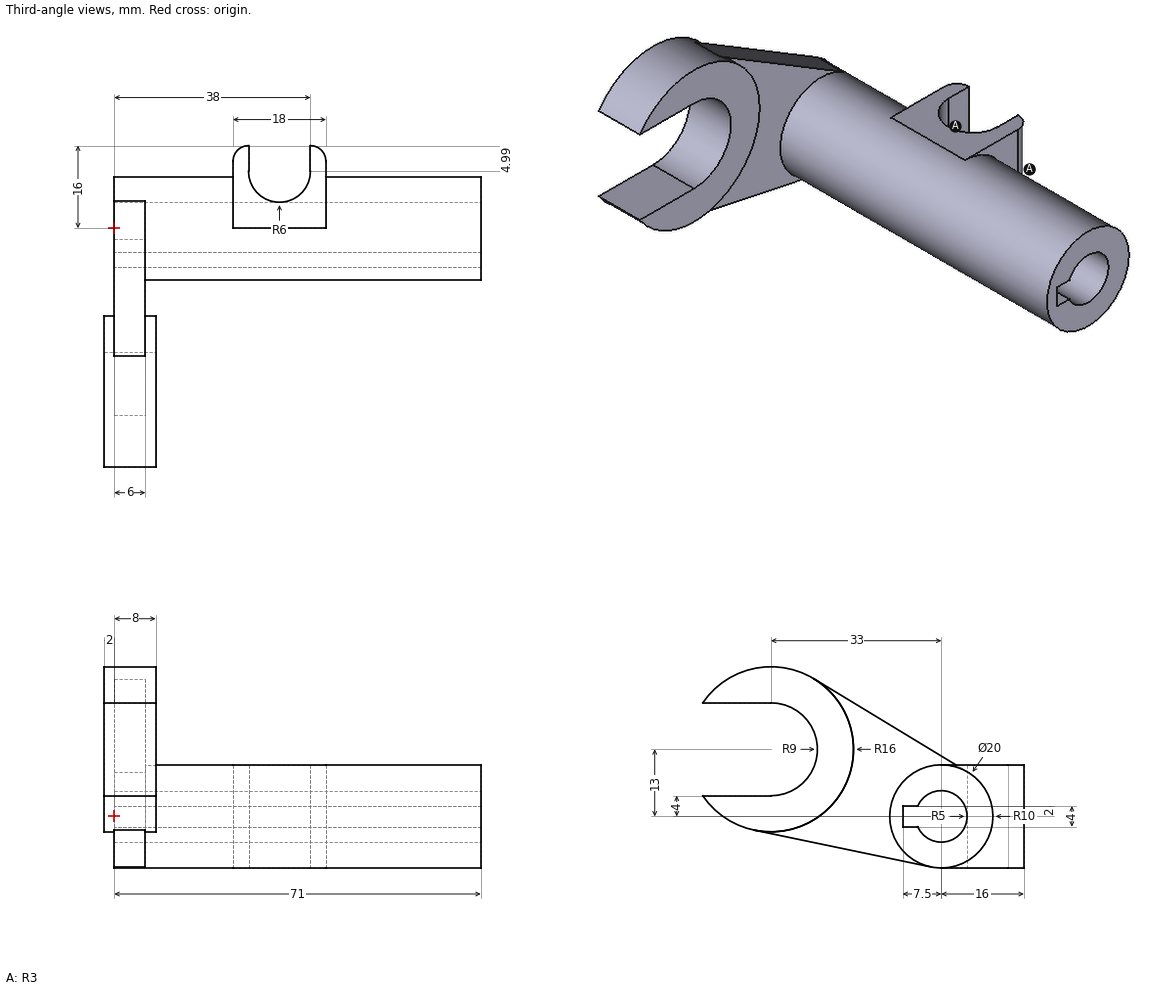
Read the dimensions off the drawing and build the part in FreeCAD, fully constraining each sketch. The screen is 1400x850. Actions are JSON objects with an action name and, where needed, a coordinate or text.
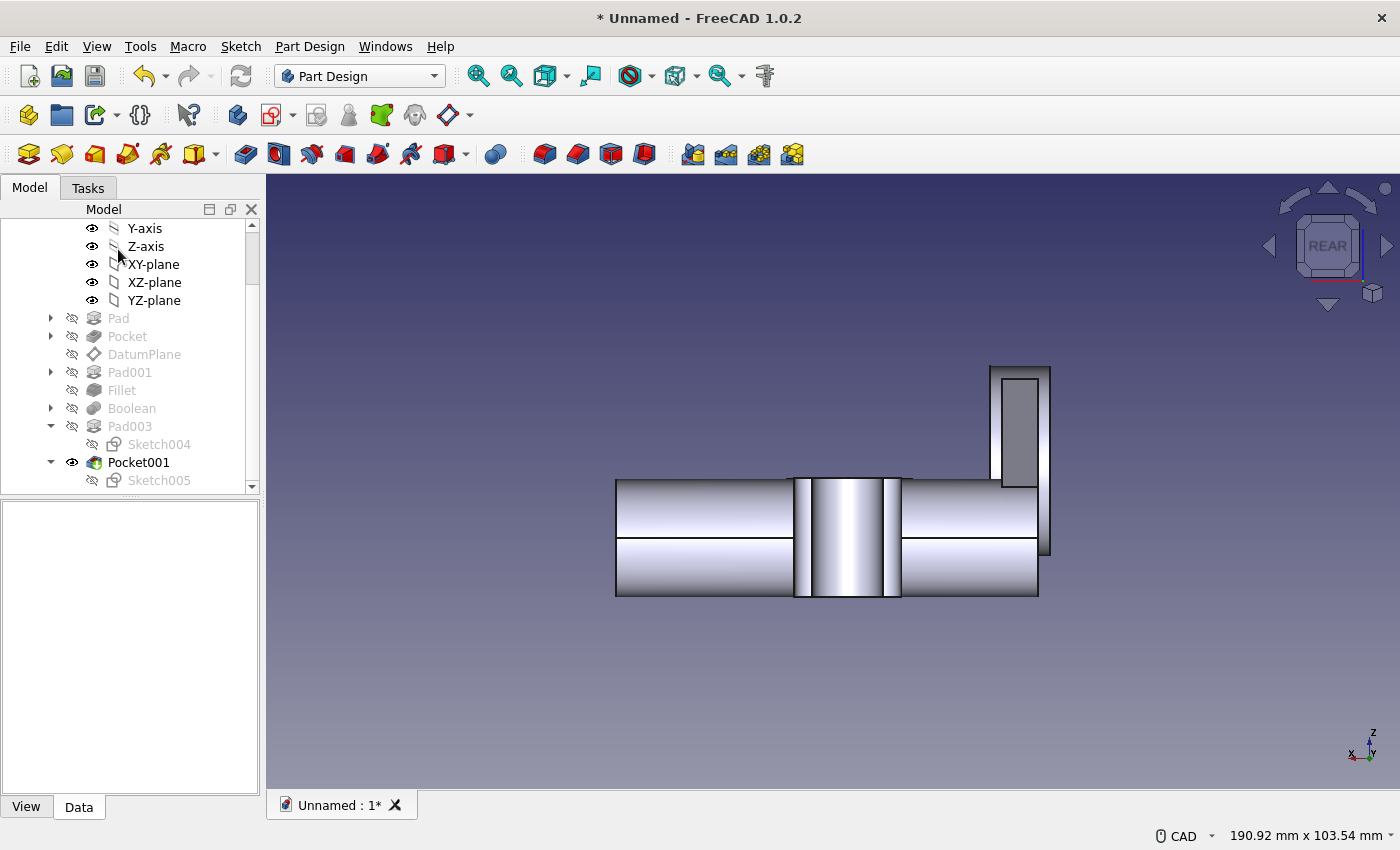
{"action": "key", "text": "0"}